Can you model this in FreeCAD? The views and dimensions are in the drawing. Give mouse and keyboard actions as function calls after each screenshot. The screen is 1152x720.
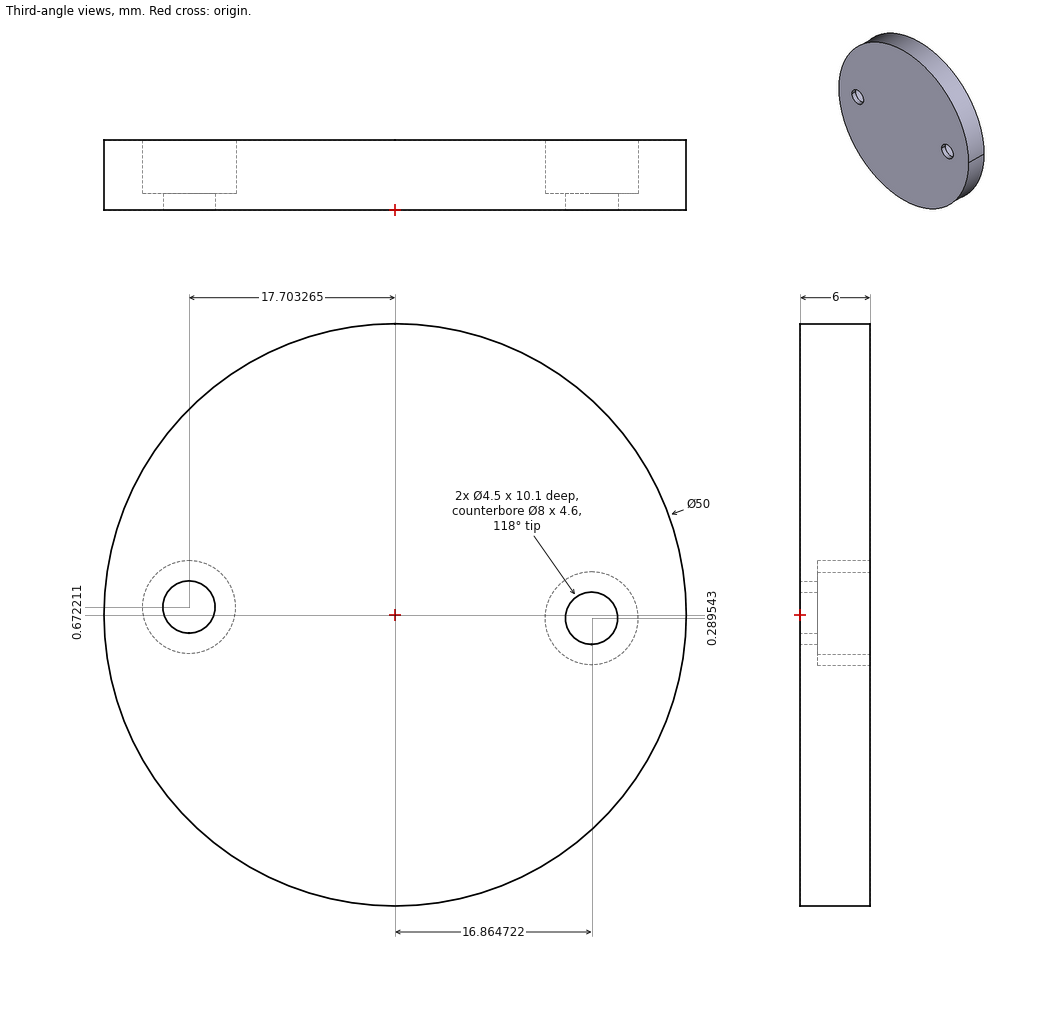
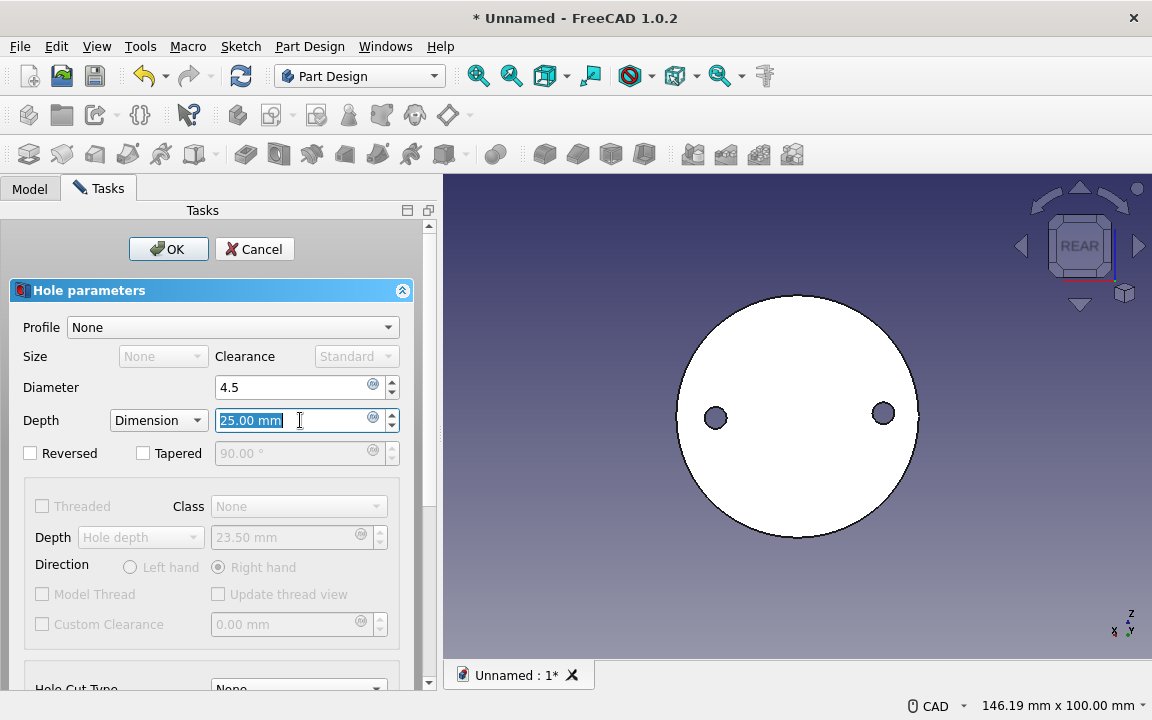
text(10.1)
key(Tab)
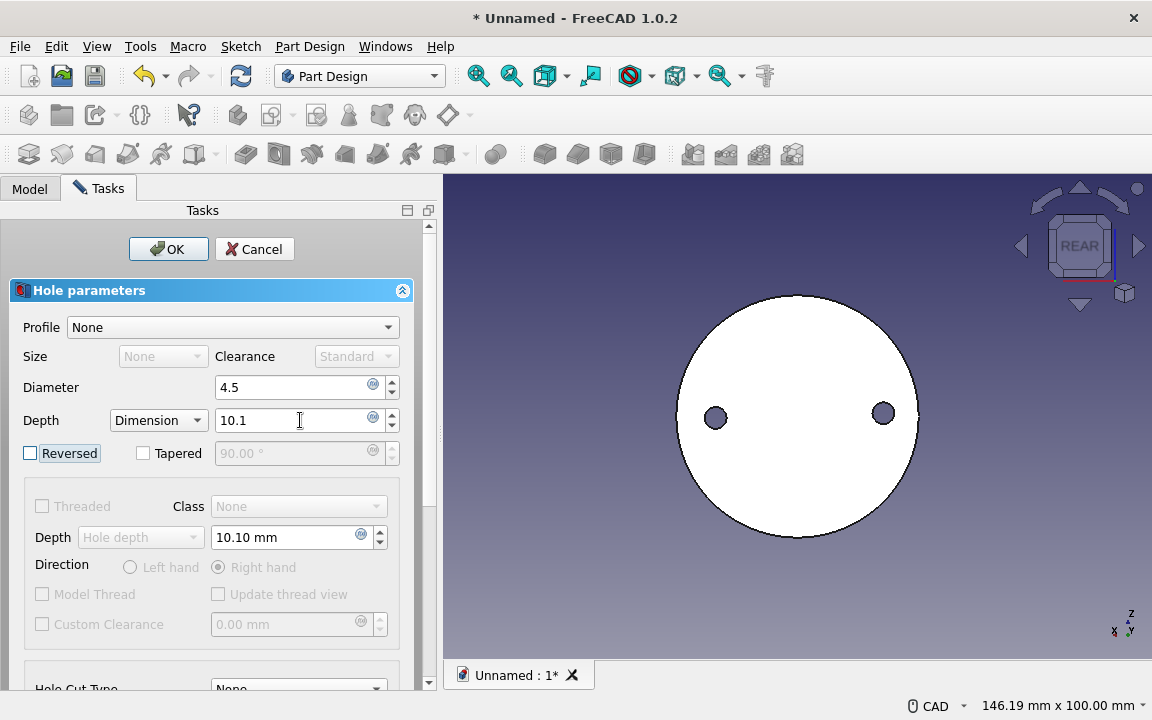
scroll(429, 455, down, 2)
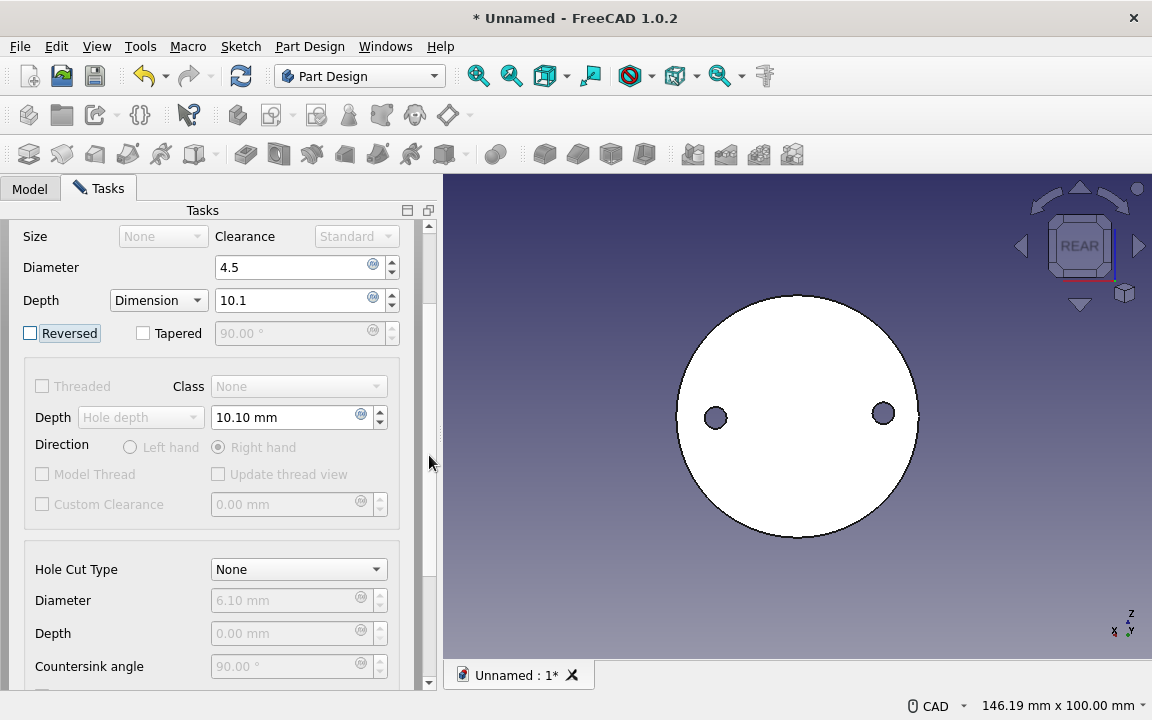
click(300, 570)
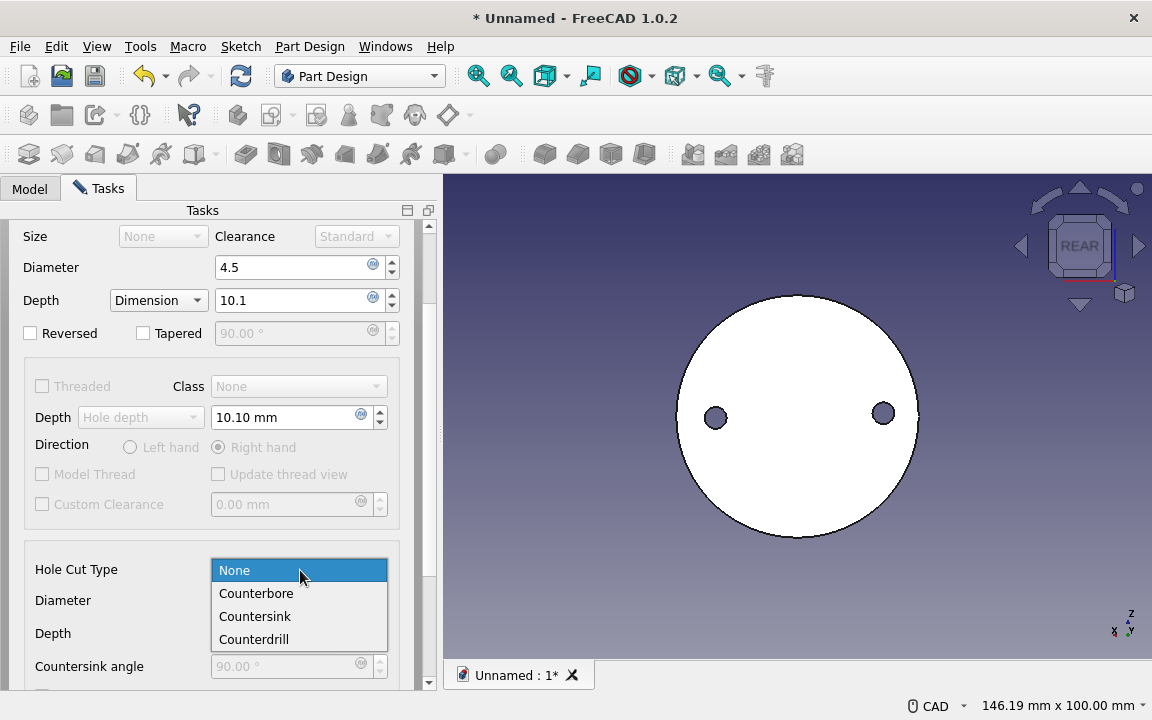
click(298, 594)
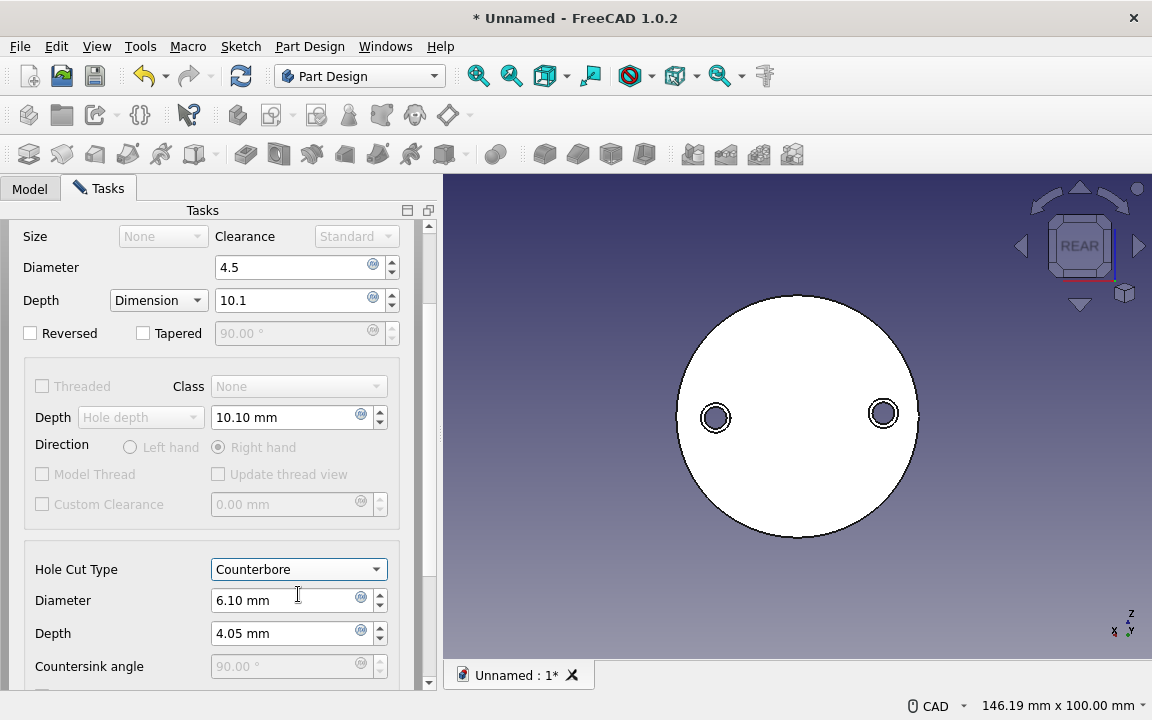
triple_click(292, 600)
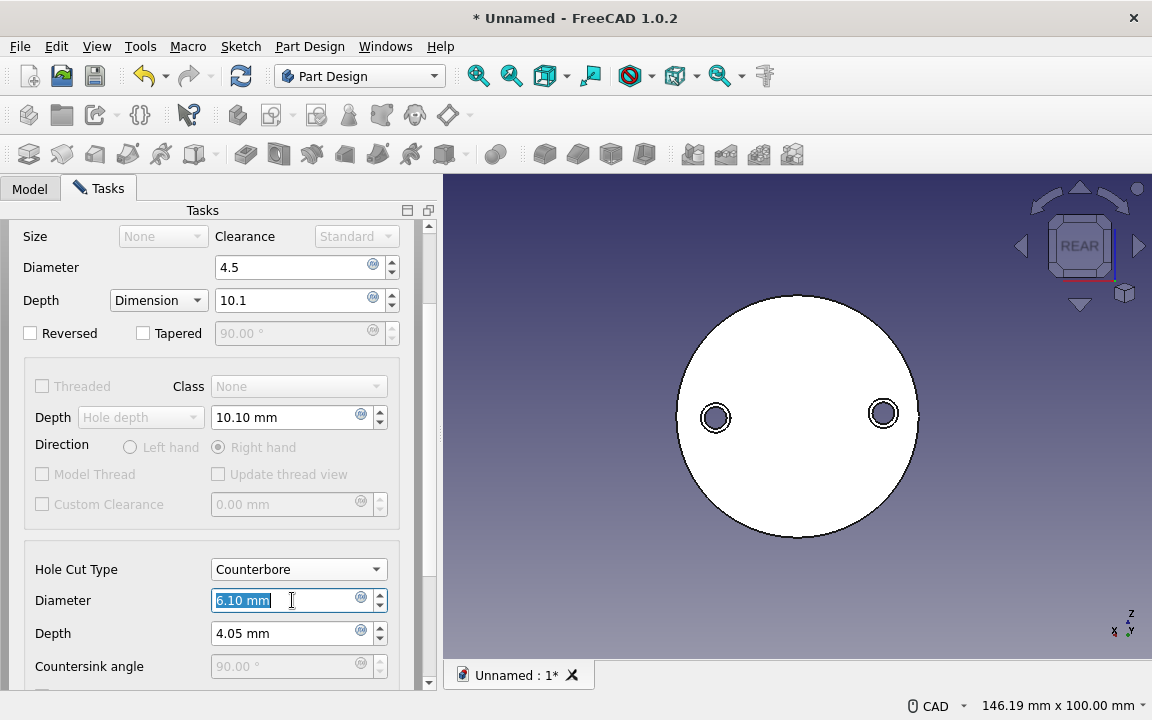
text(8)
key(Tab)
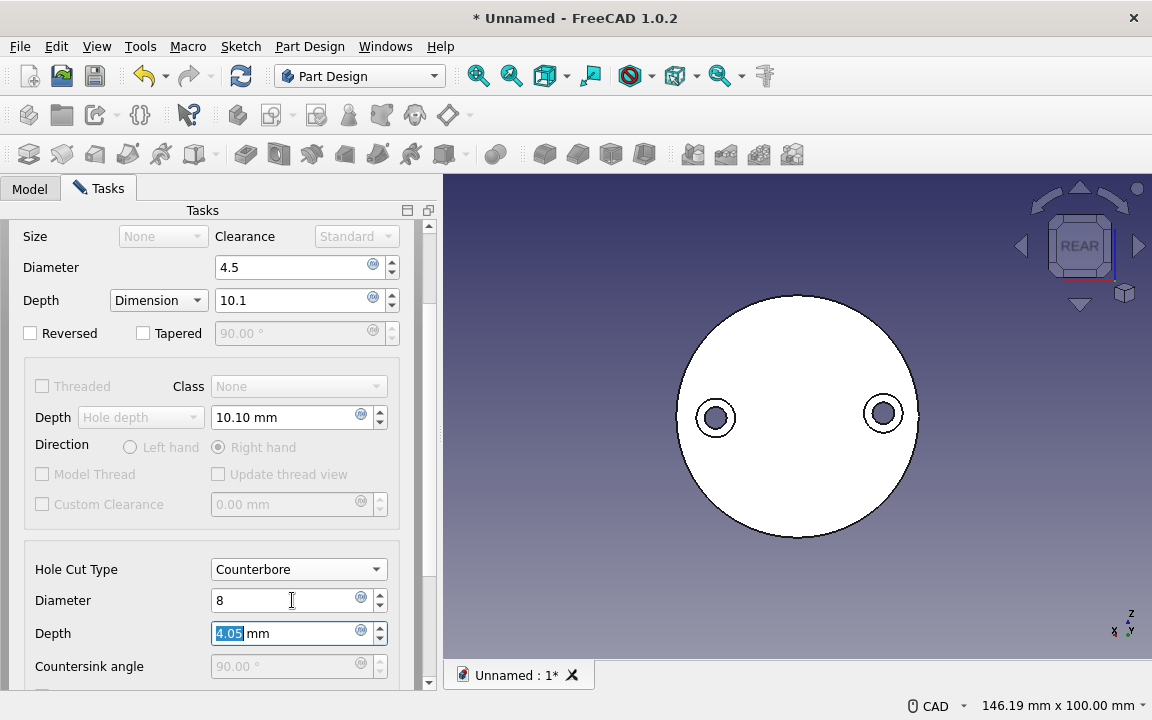
text(4.6)
key(Tab)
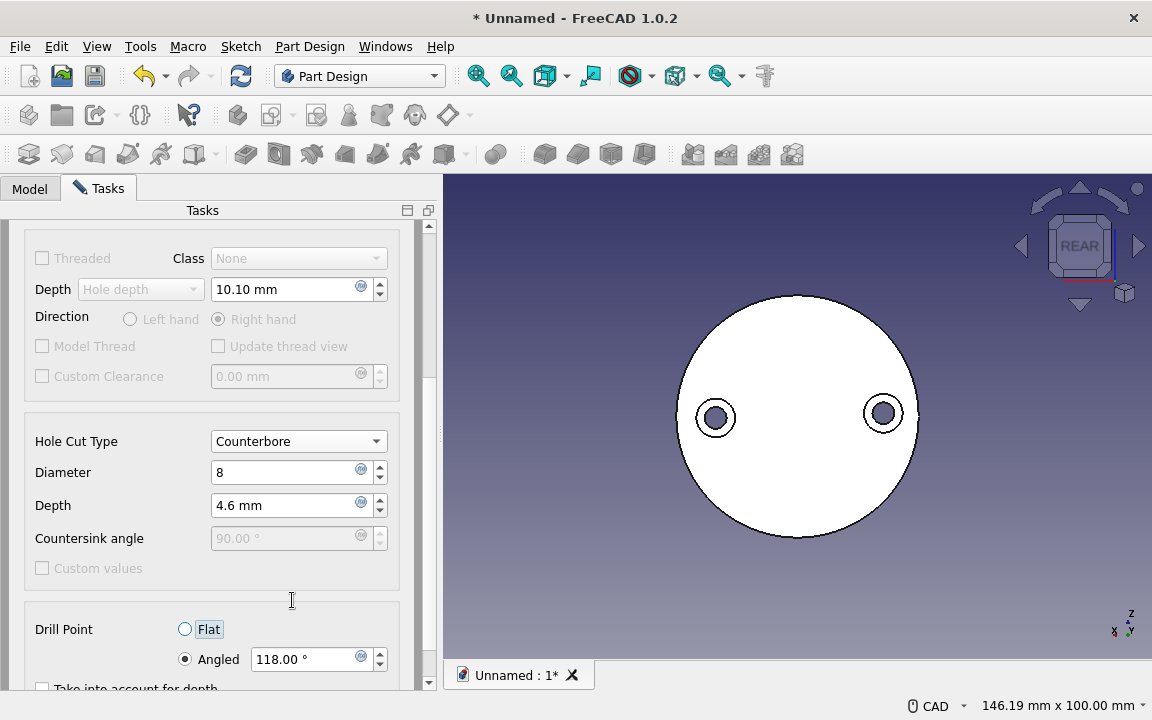
scroll(429, 455, up, 5)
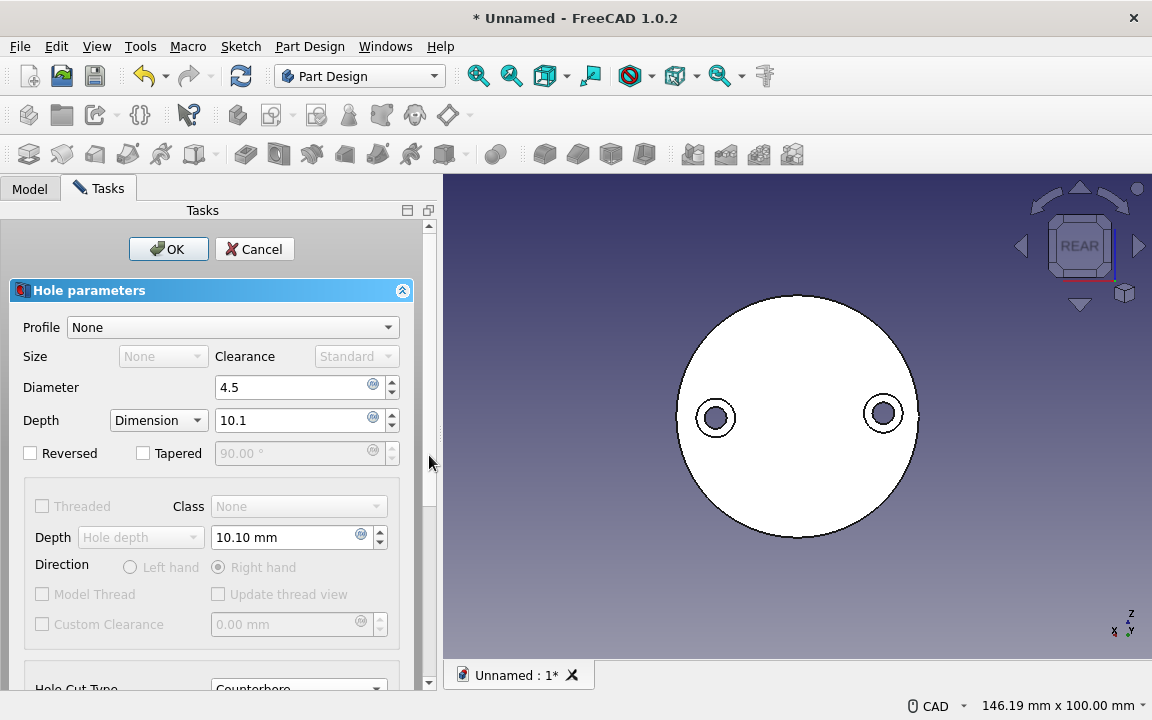
click(169, 249)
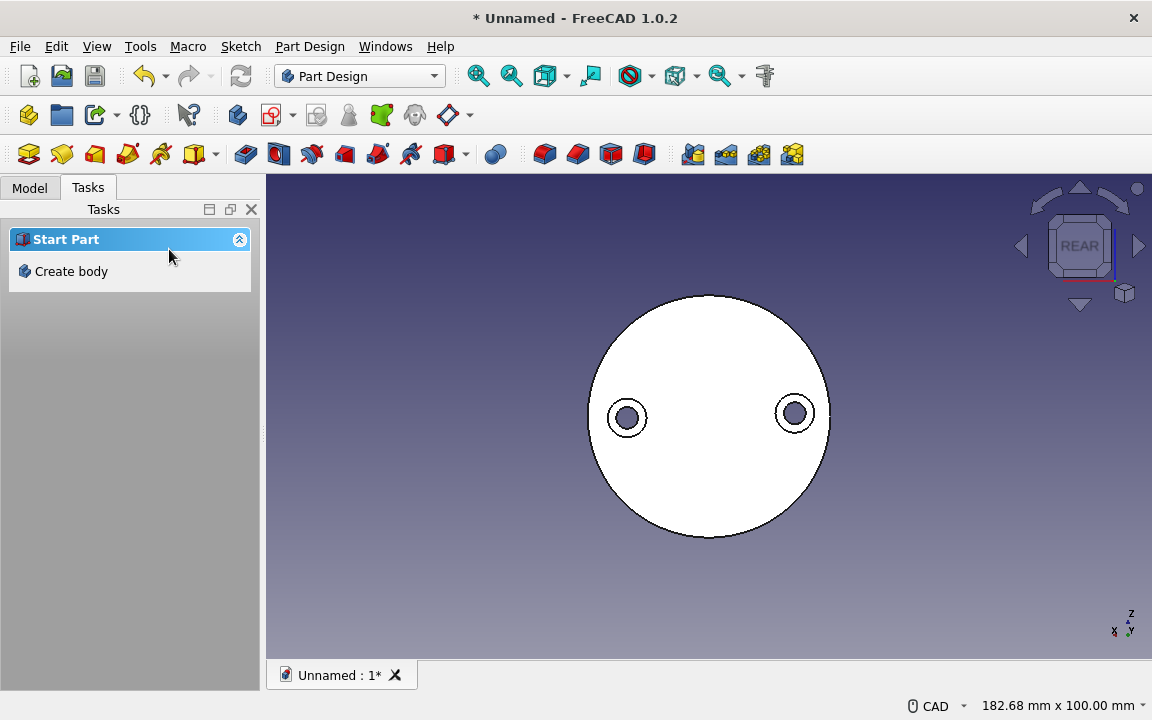
key(0)